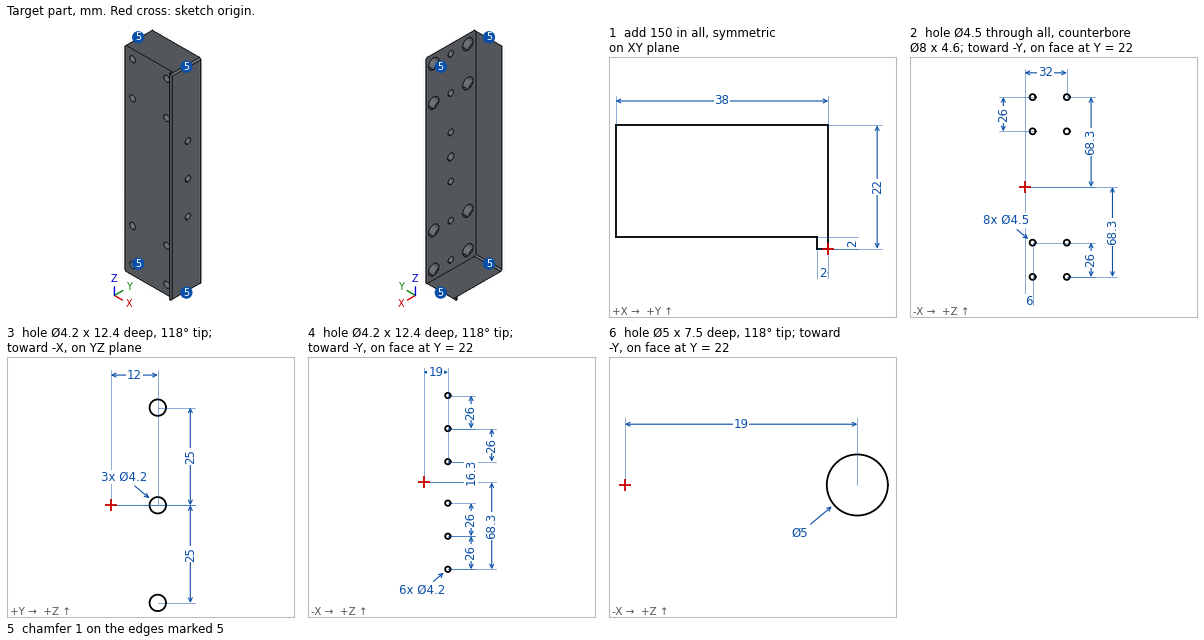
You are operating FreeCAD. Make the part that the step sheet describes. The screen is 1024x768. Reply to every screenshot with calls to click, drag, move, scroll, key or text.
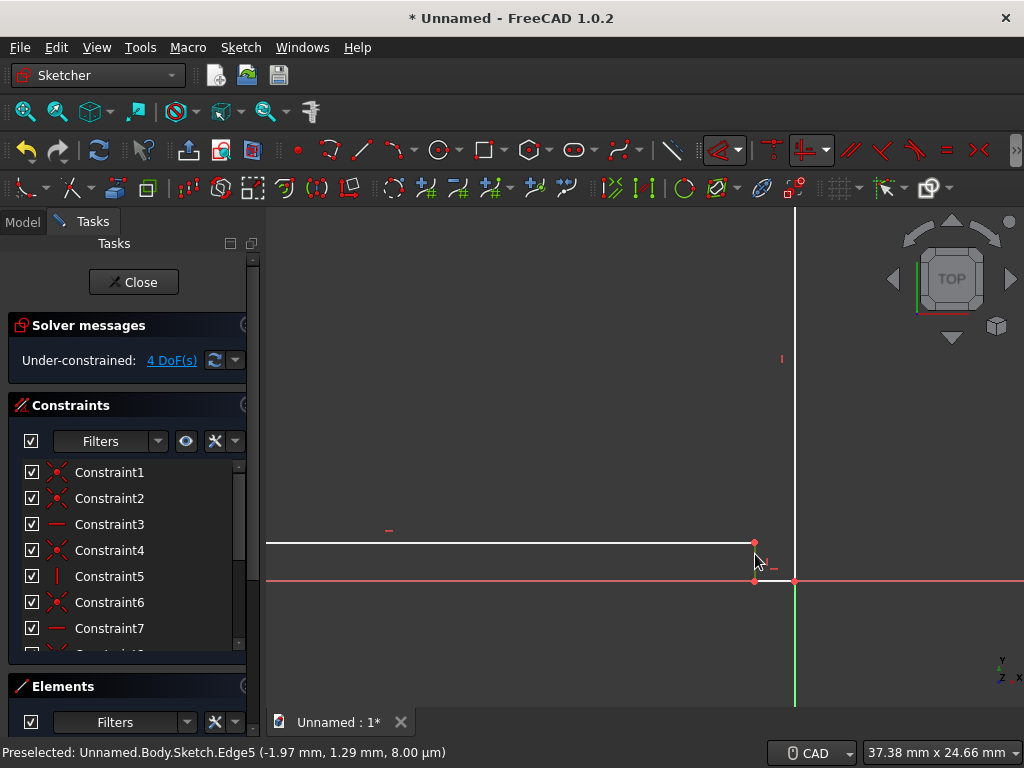
key(i)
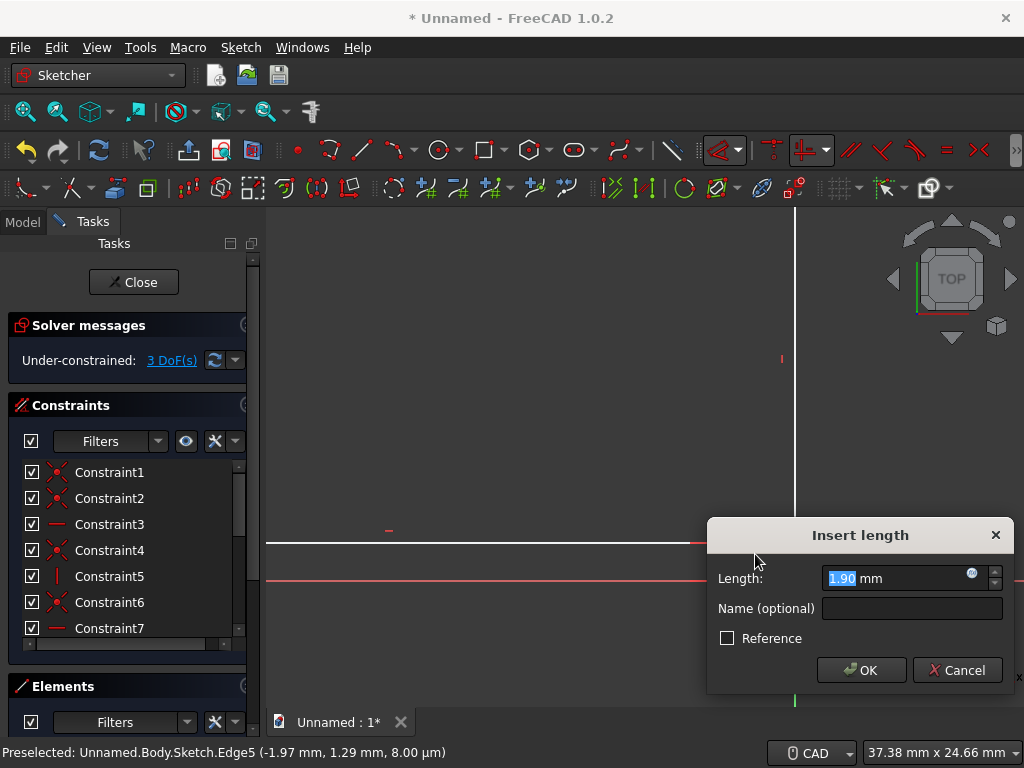
text(2)
key(Return)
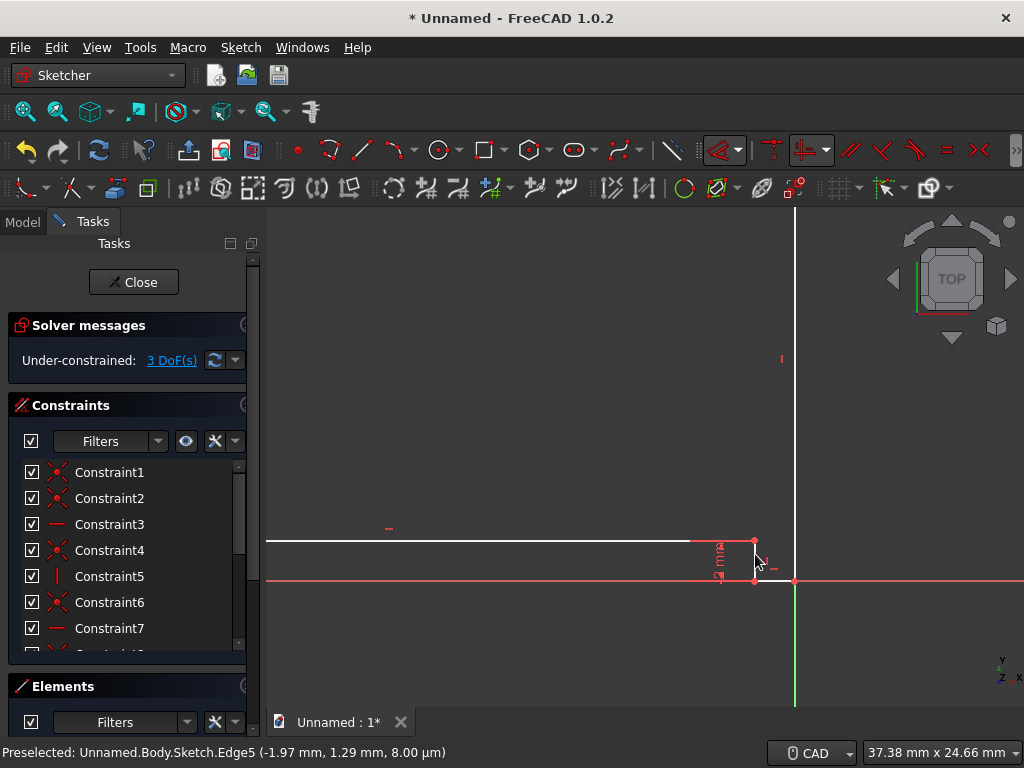
click(767, 581)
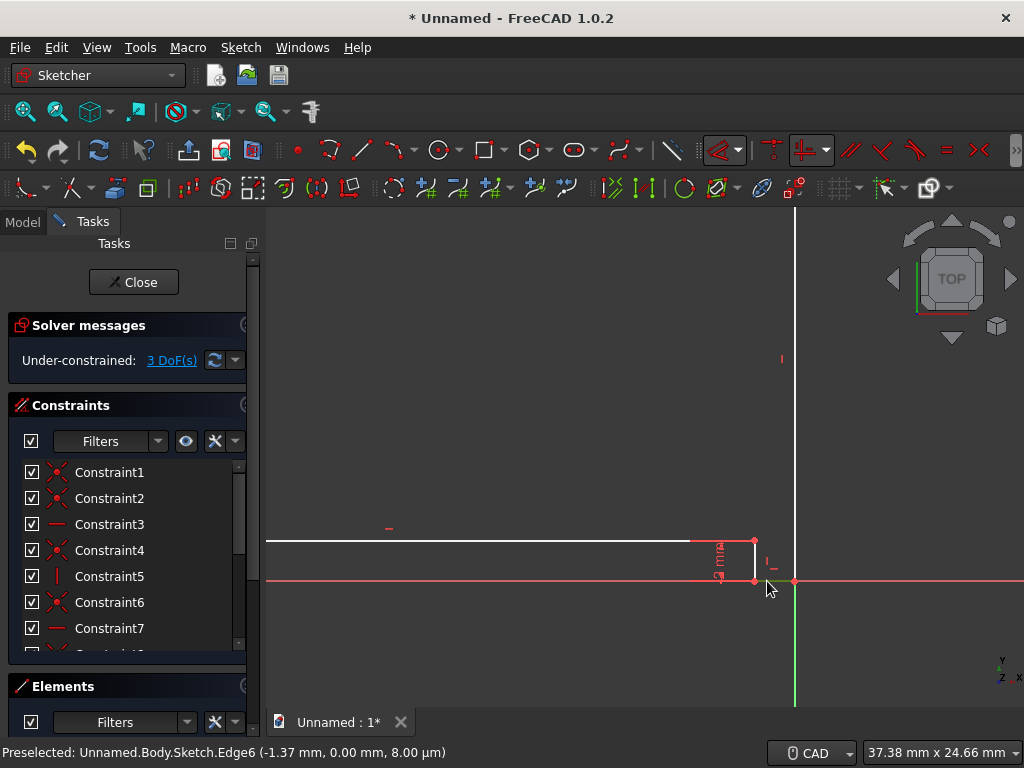
key(l)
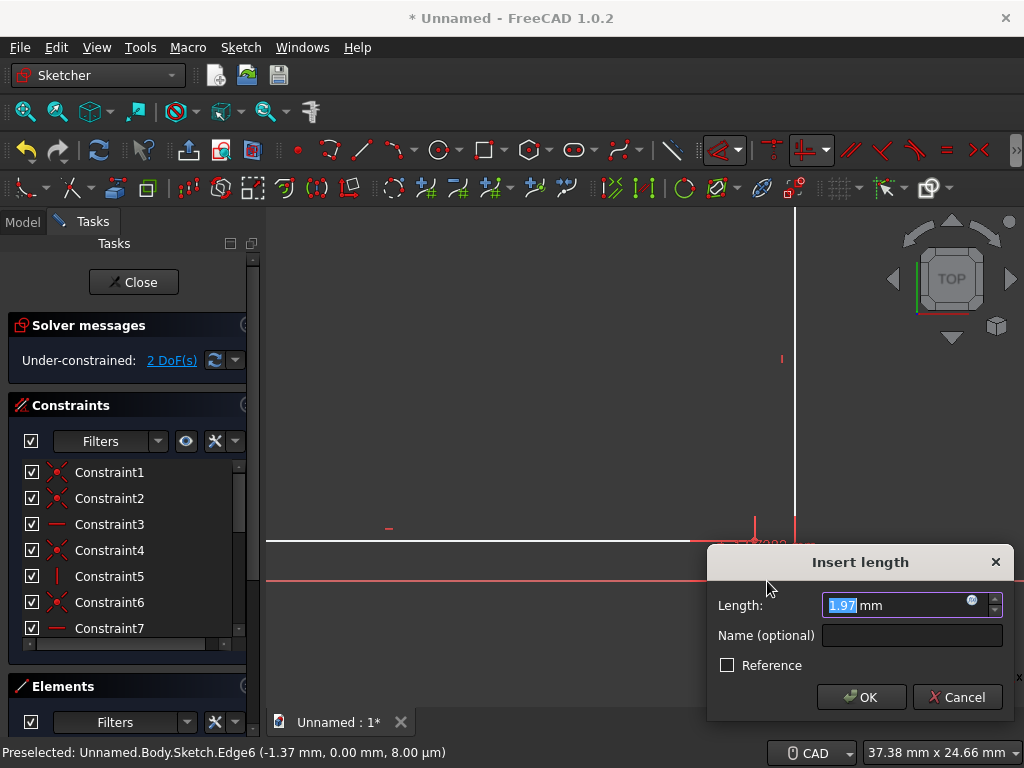
text(2)
key(Return)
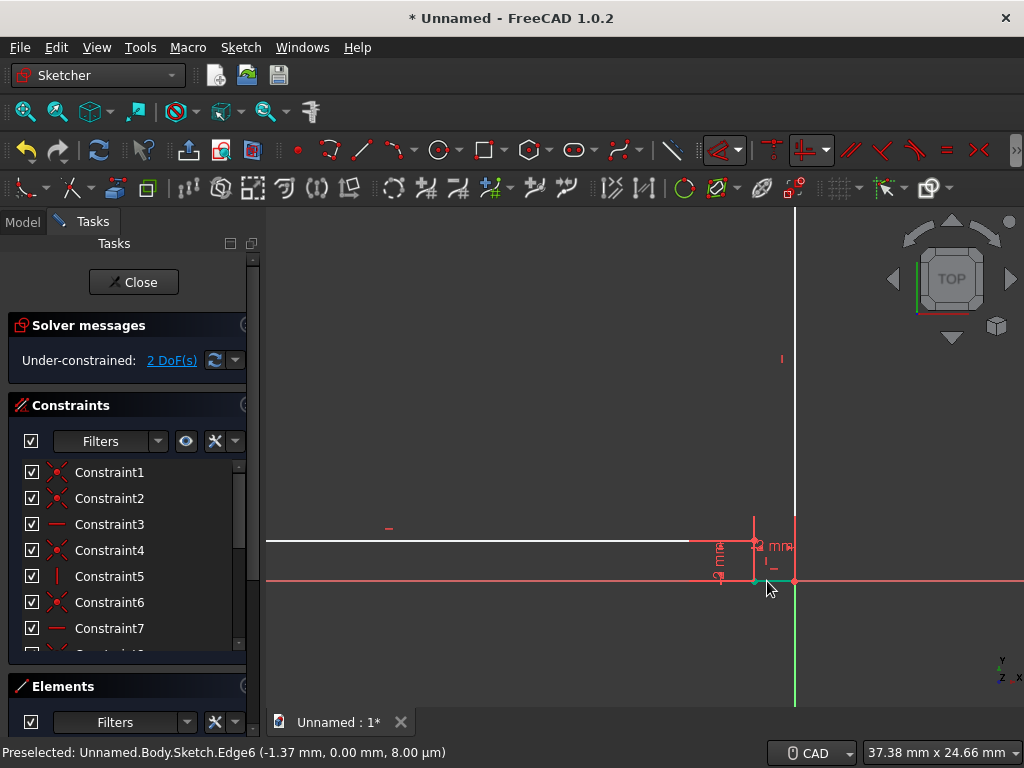
click(795, 448)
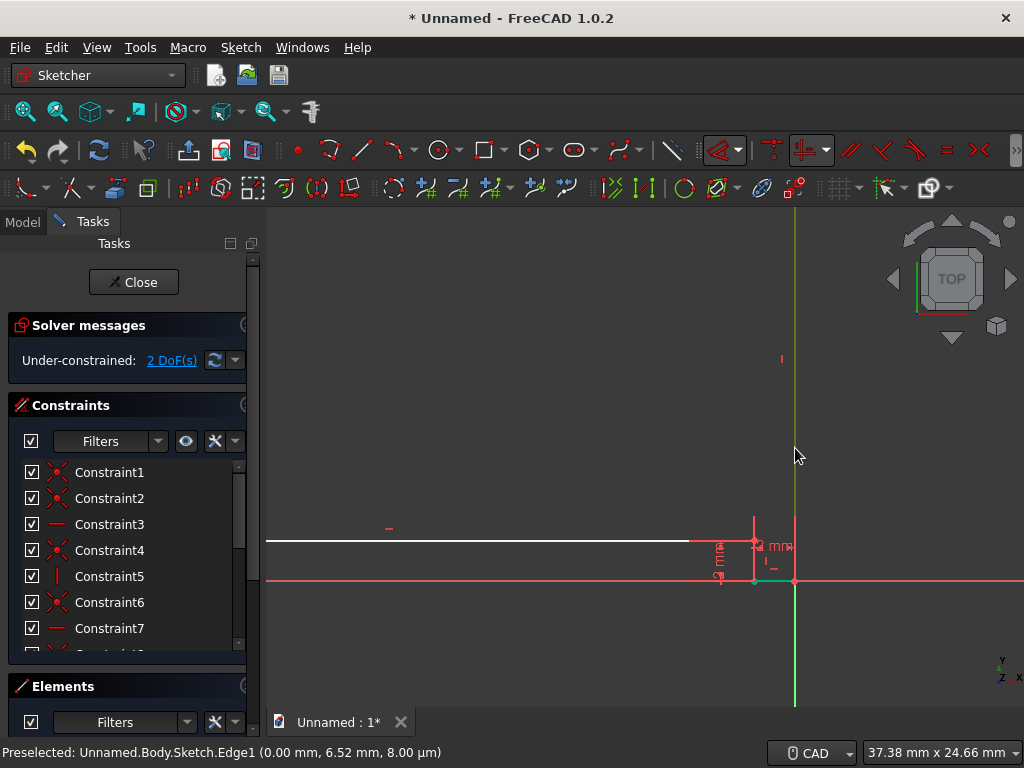
key(i)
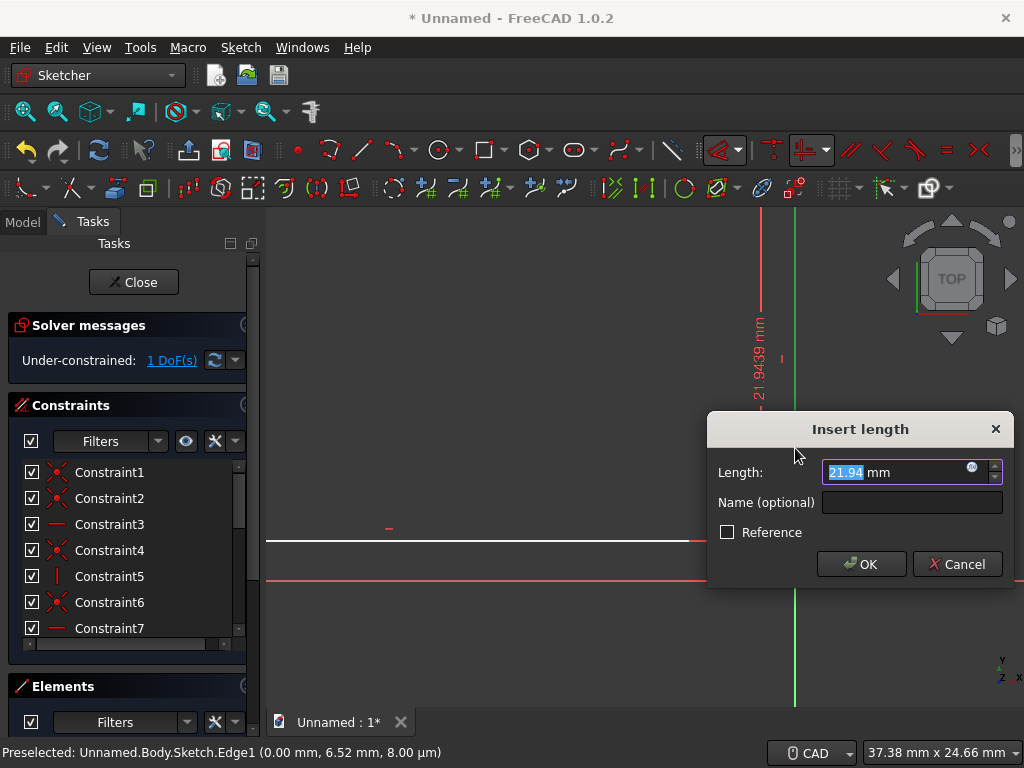
text(22)
key(Return)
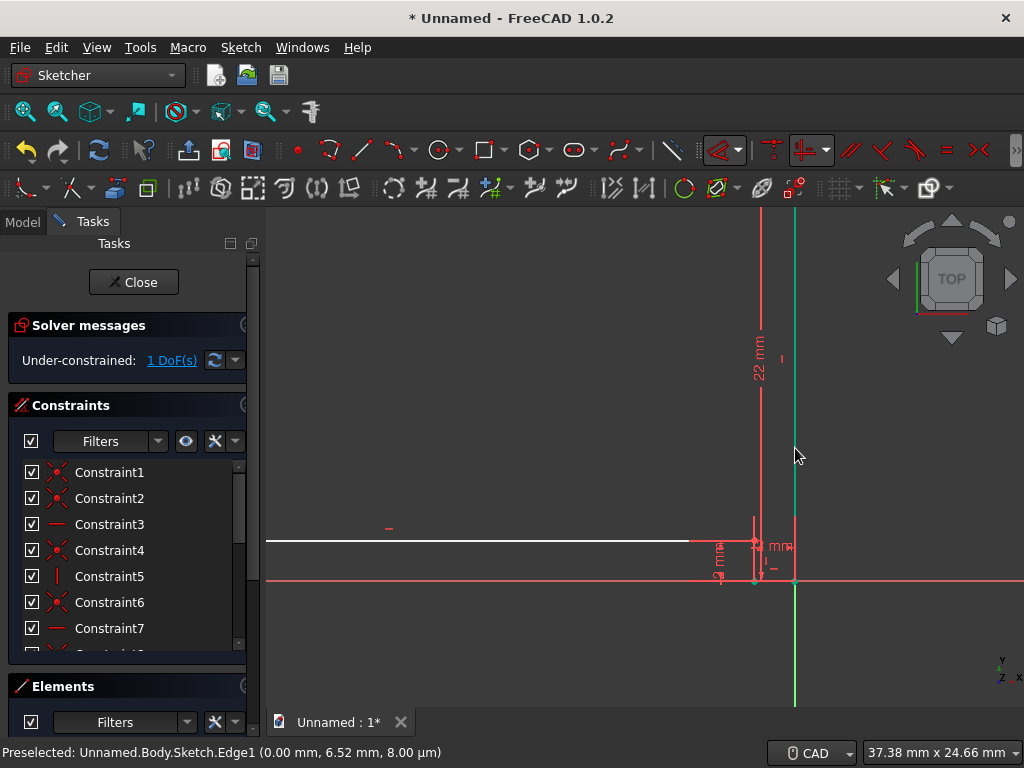
scroll(780, 577, down, 3)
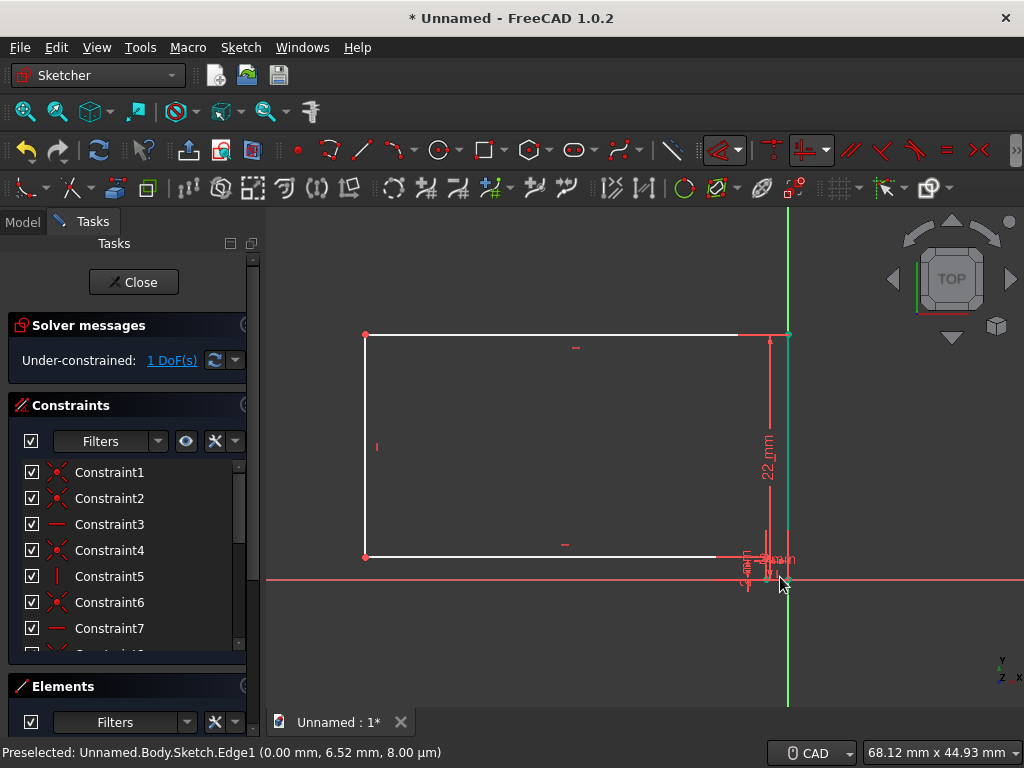
click(662, 335)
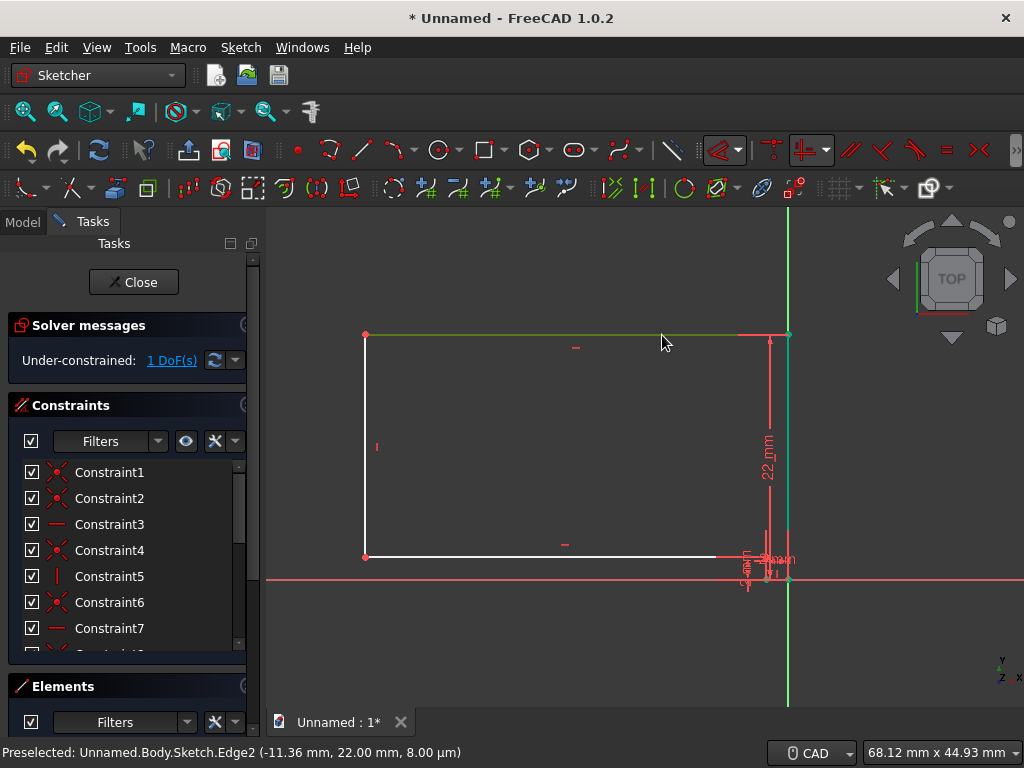
key(l)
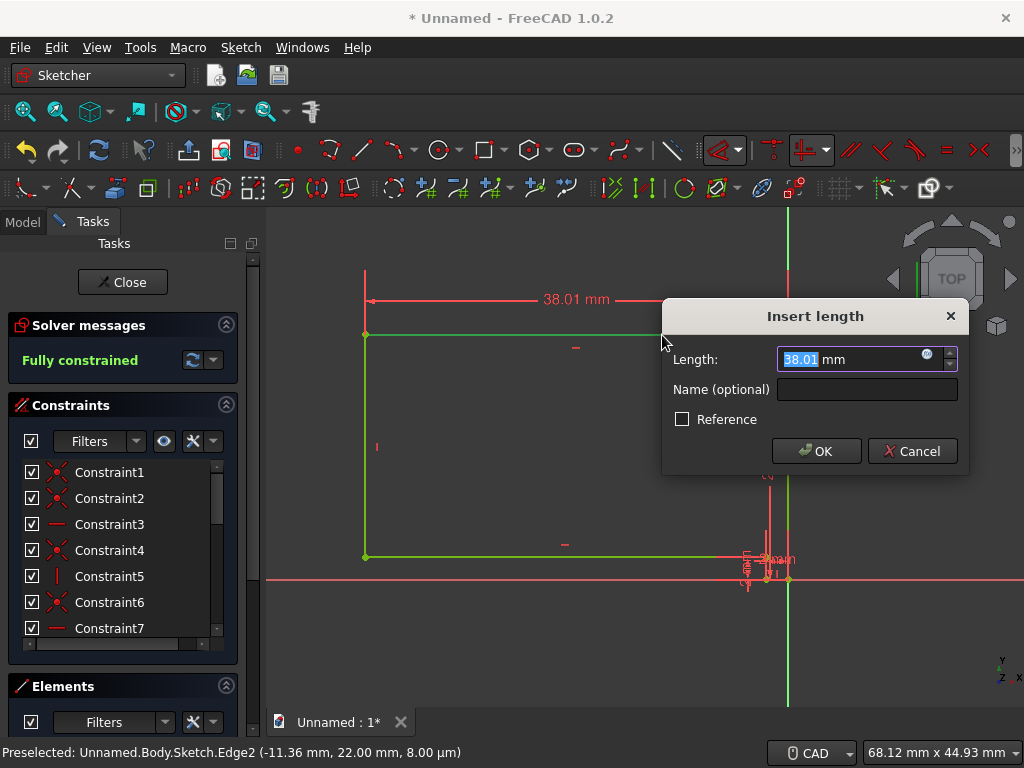
text(38)
key(Return)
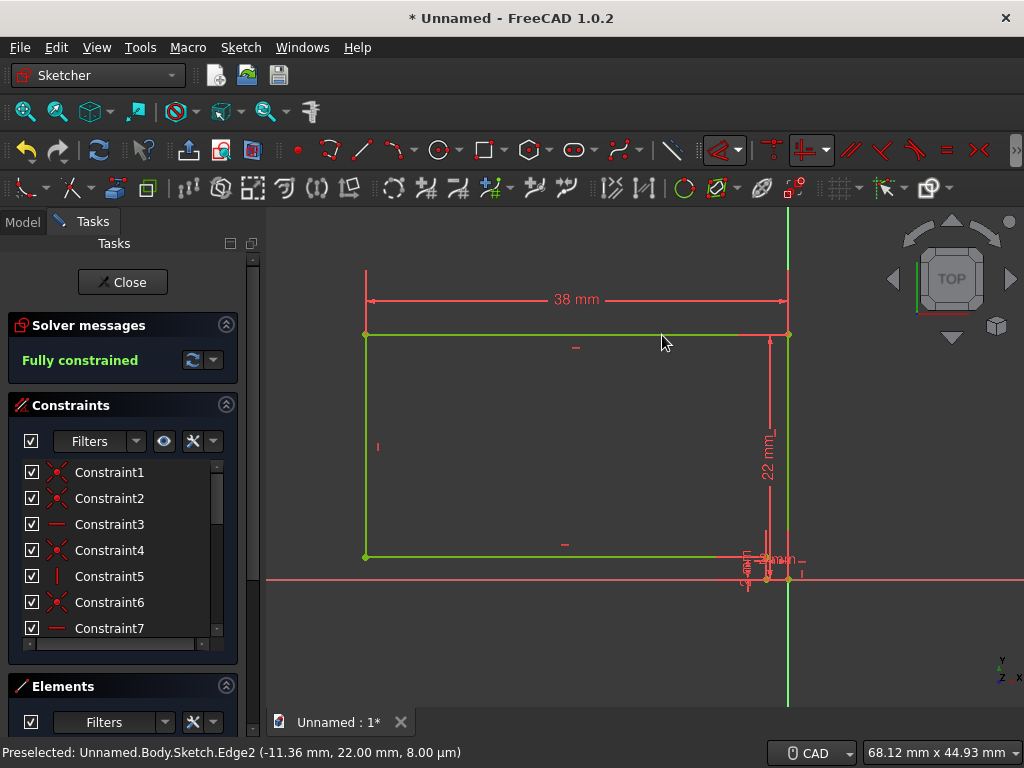
click(123, 282)